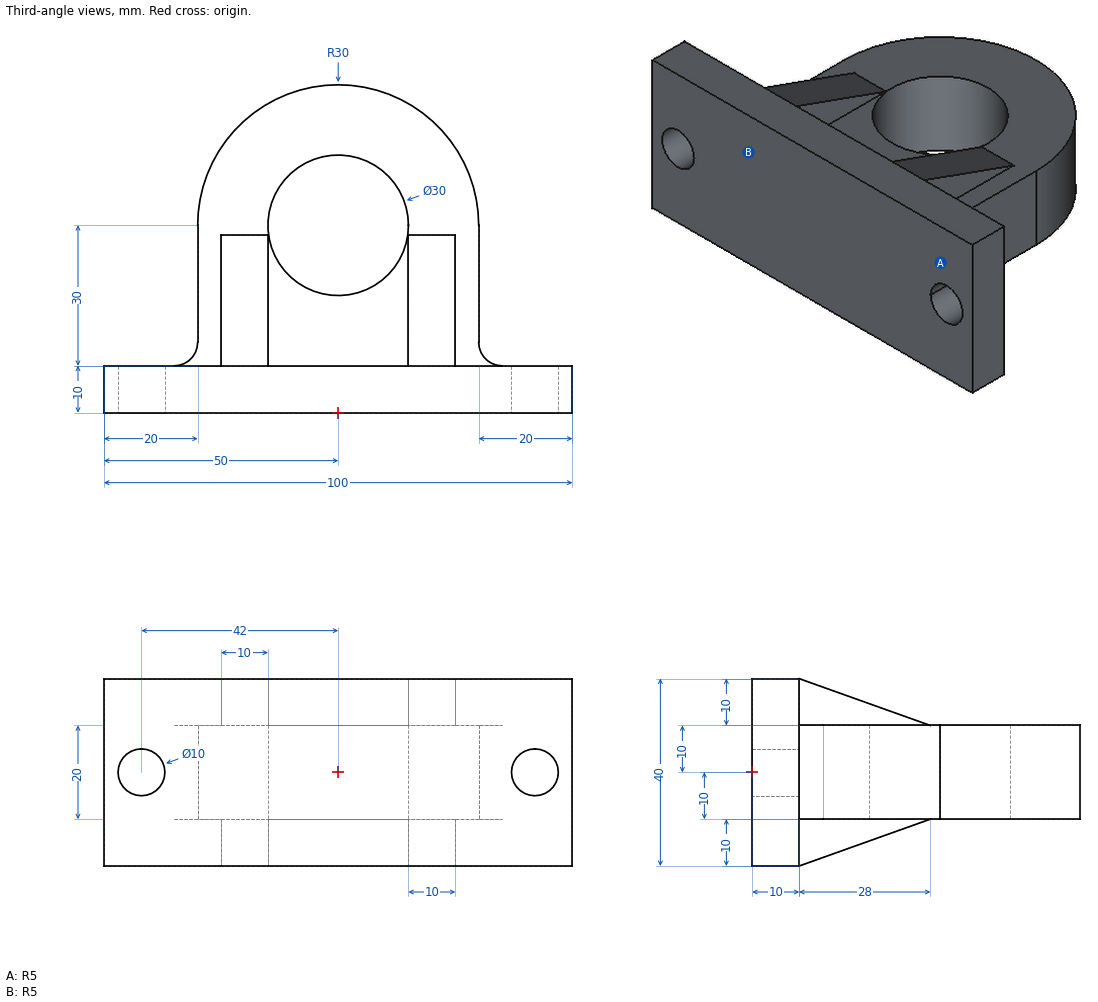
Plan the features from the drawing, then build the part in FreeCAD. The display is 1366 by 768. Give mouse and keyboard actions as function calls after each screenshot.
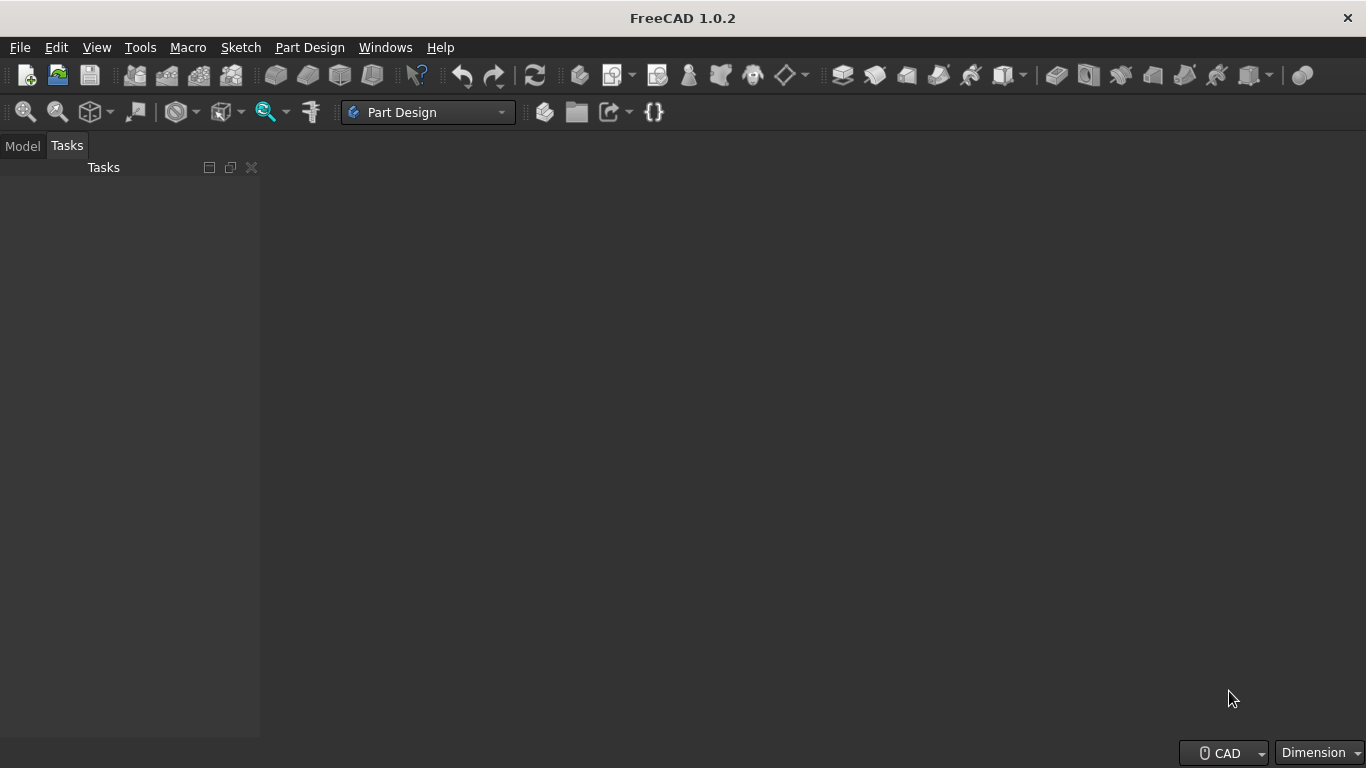
click(26, 76)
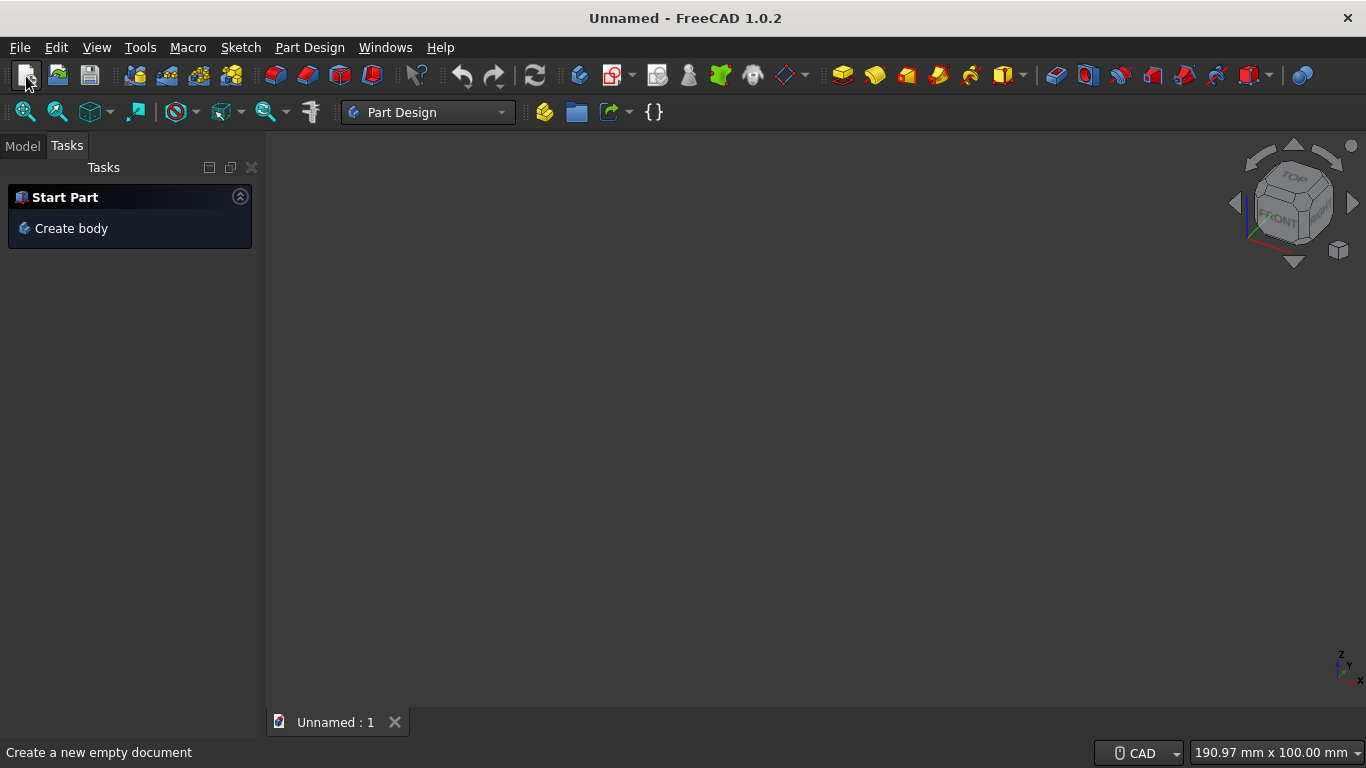
click(612, 76)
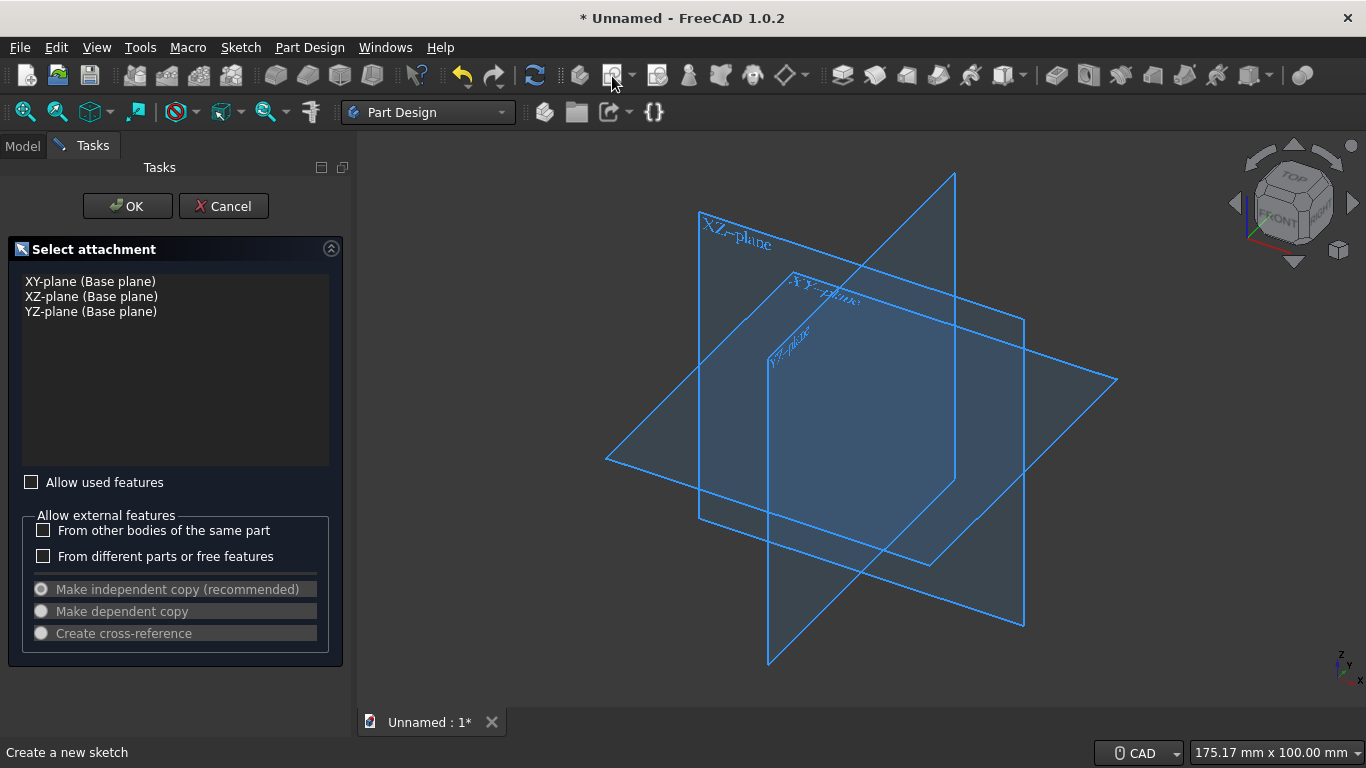
click(82, 282)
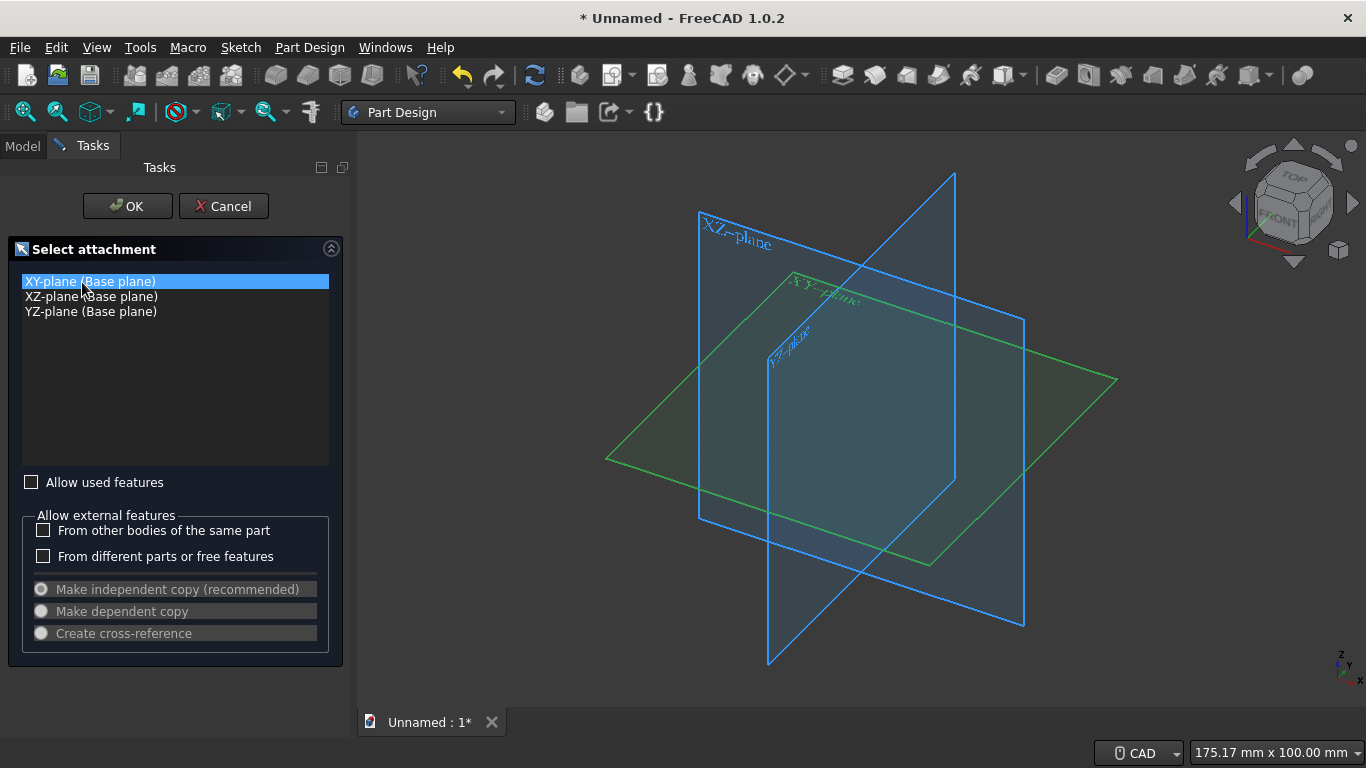
click(128, 206)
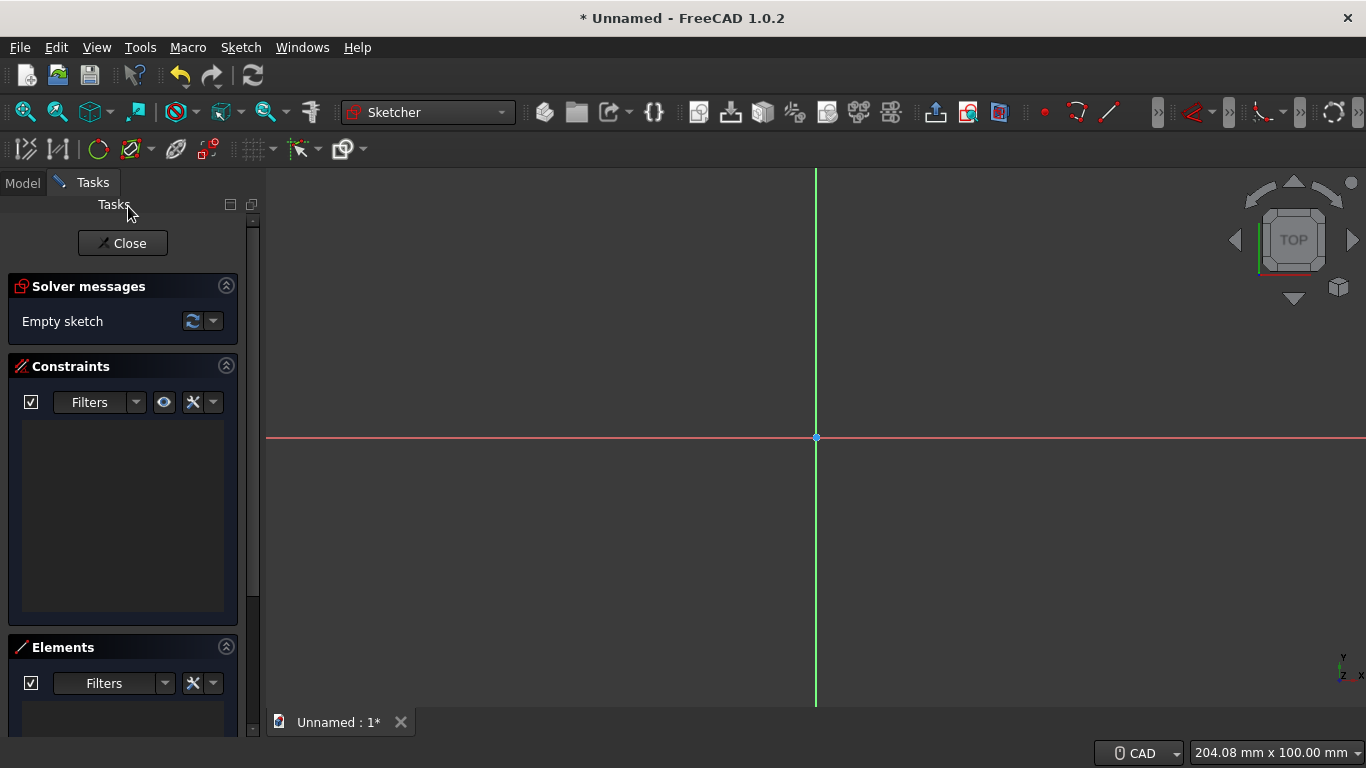
key(g)
key(r)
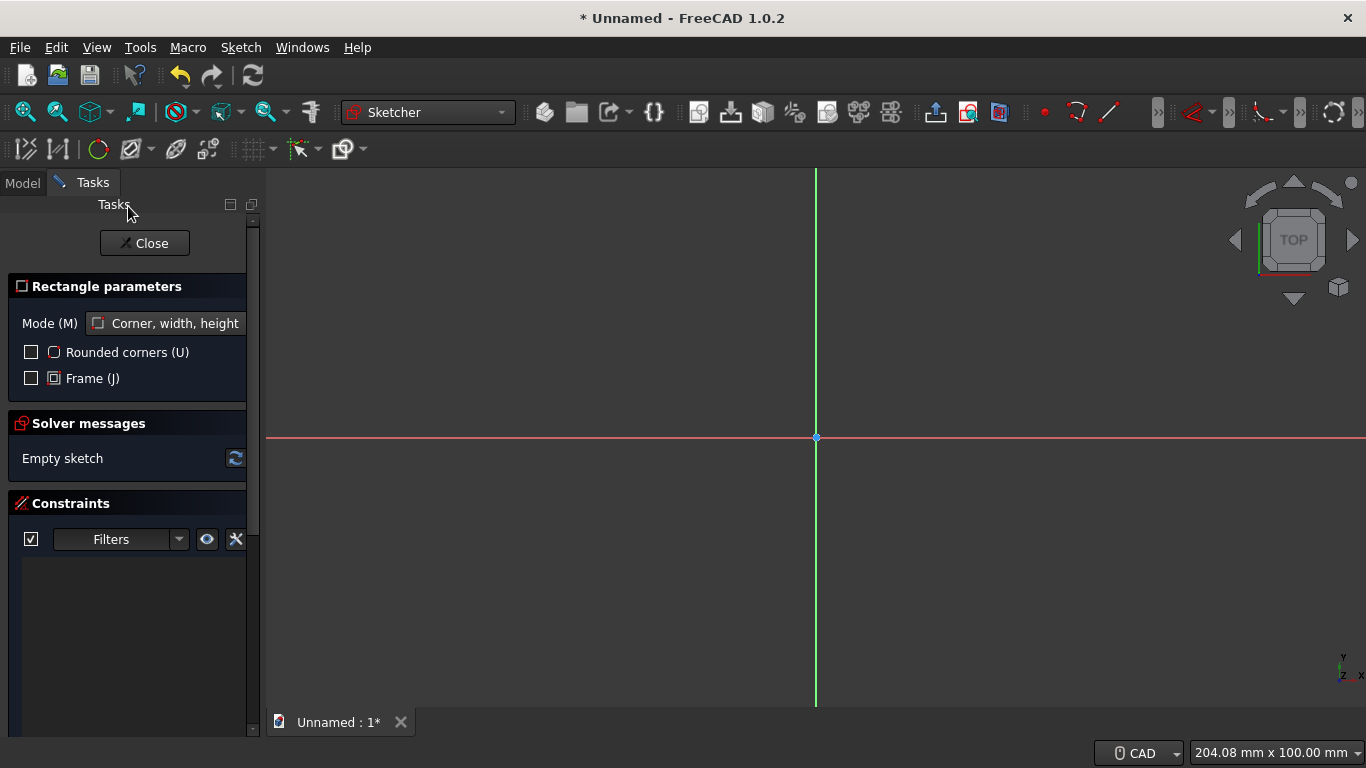
click(546, 384)
click(1086, 438)
key(Escape)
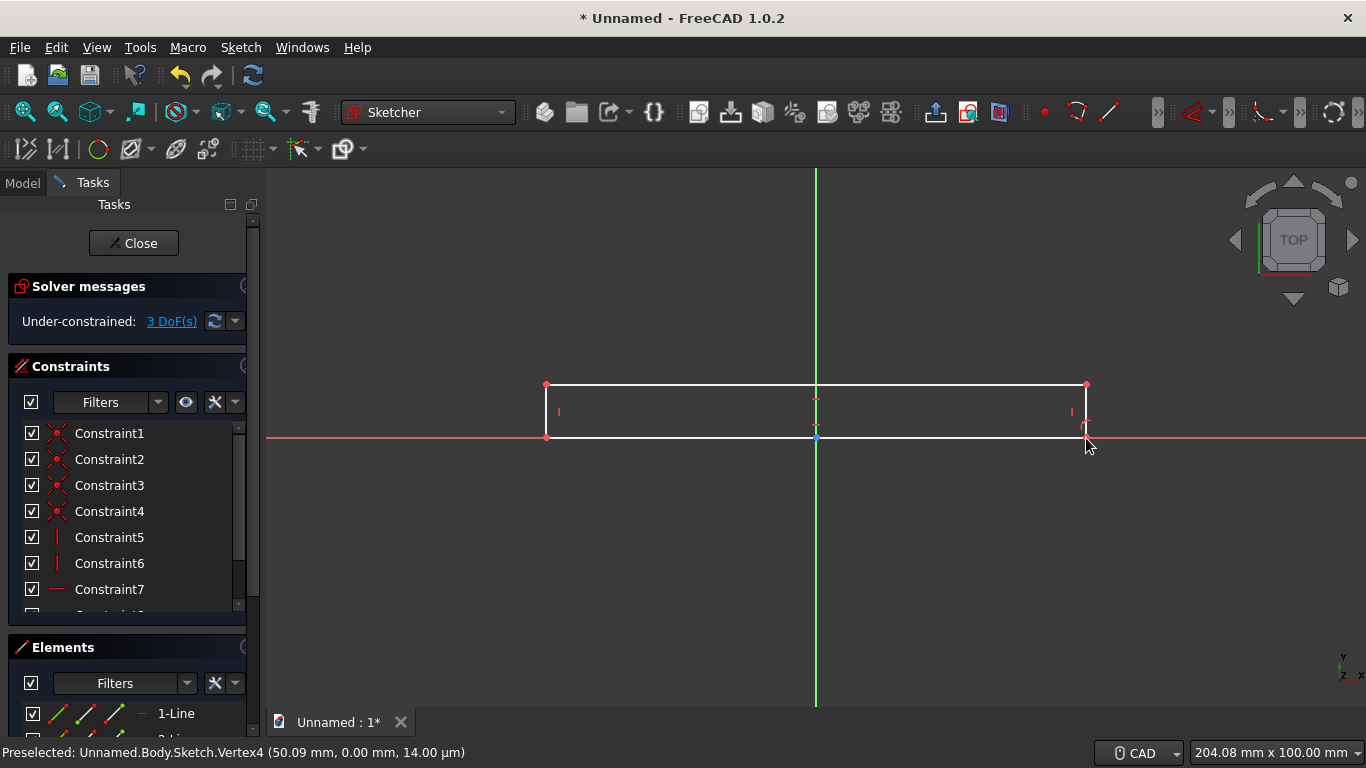
key(d)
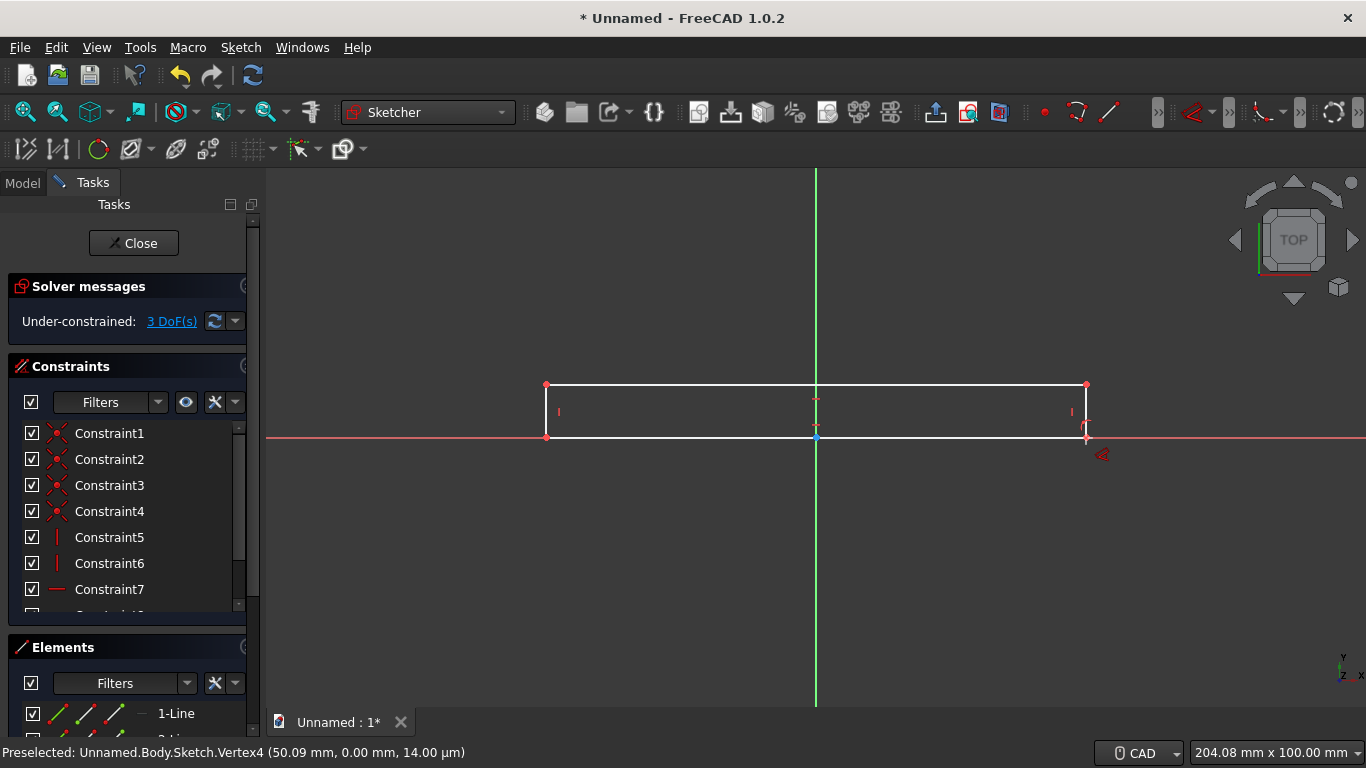
click(546, 401)
click(512, 411)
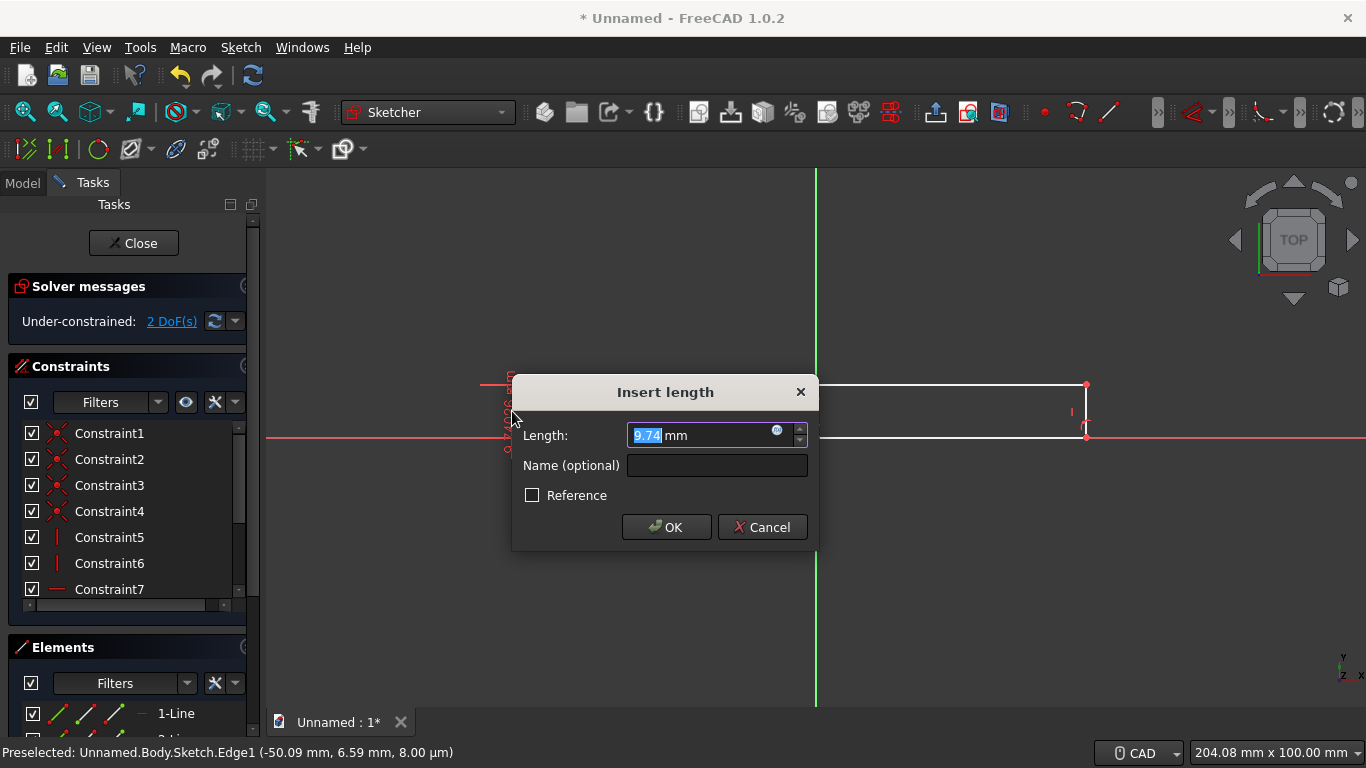
text(10)
key(Return)